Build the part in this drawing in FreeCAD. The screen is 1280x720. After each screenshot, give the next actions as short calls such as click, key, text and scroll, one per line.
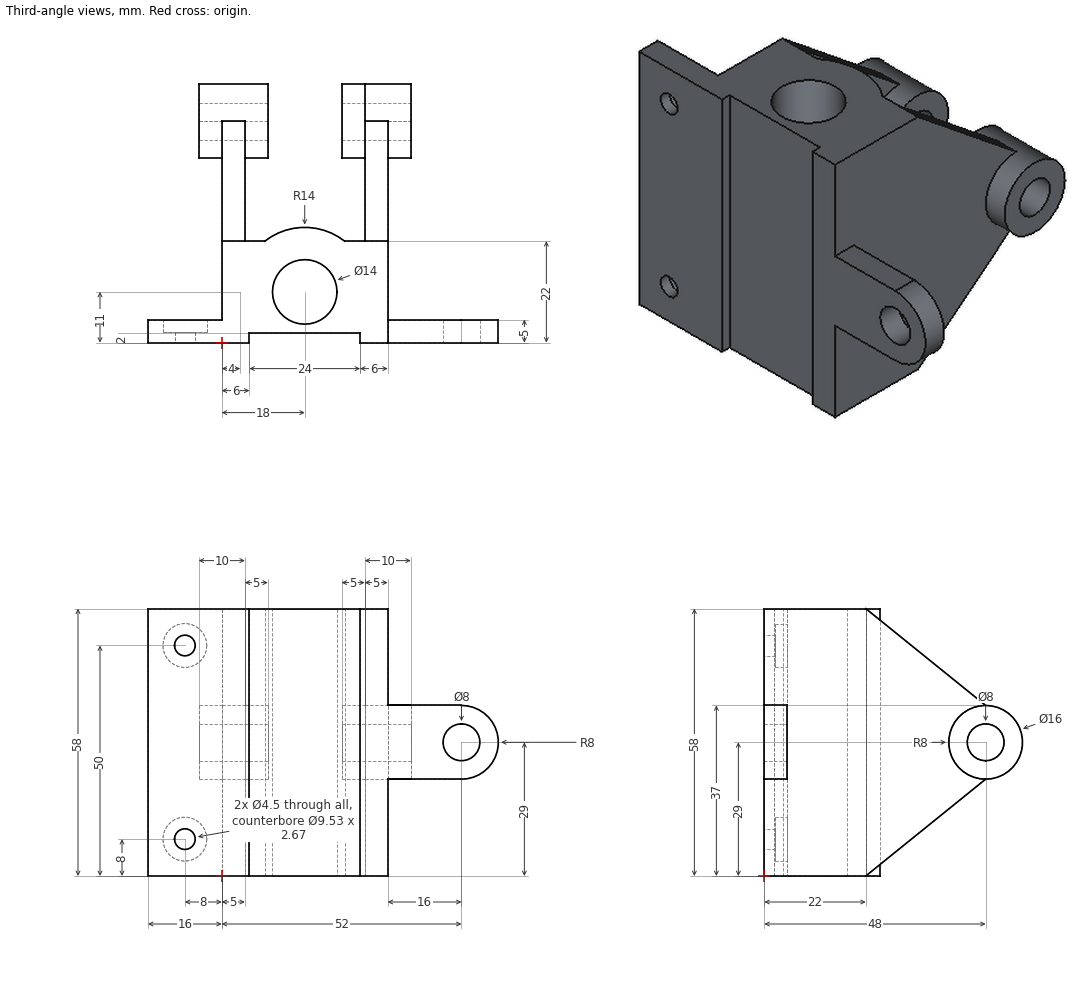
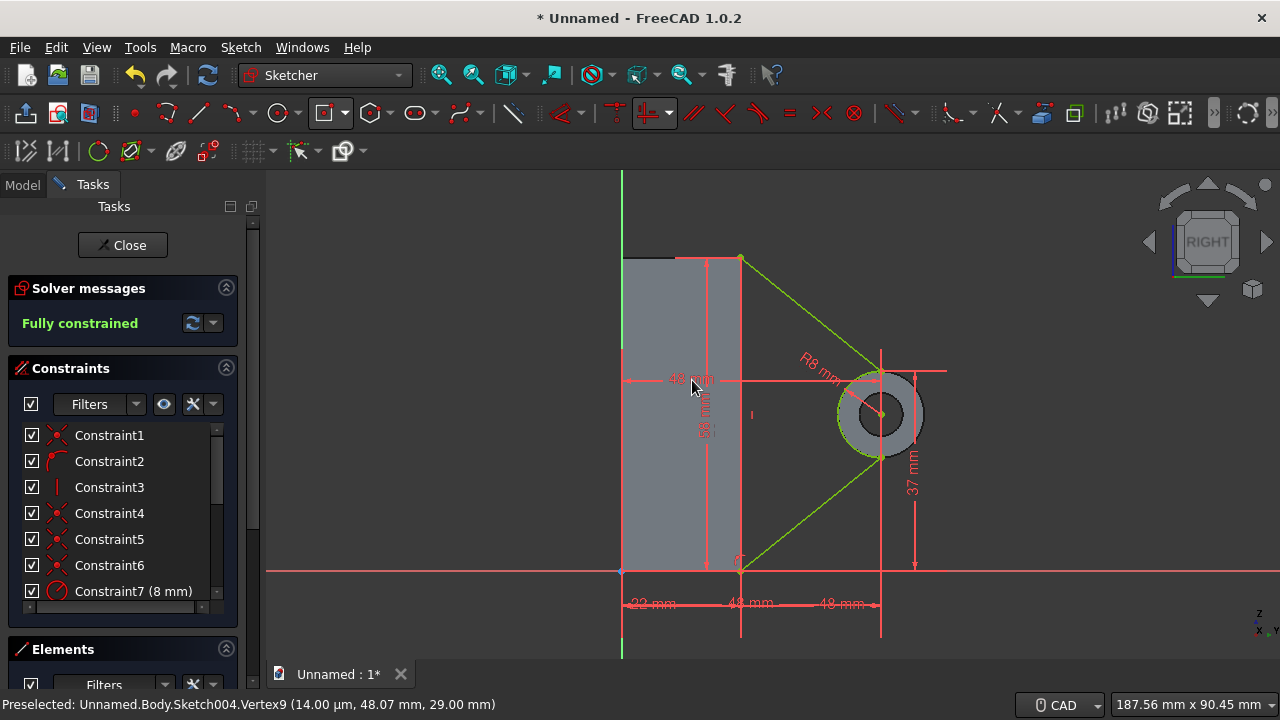
click(123, 245)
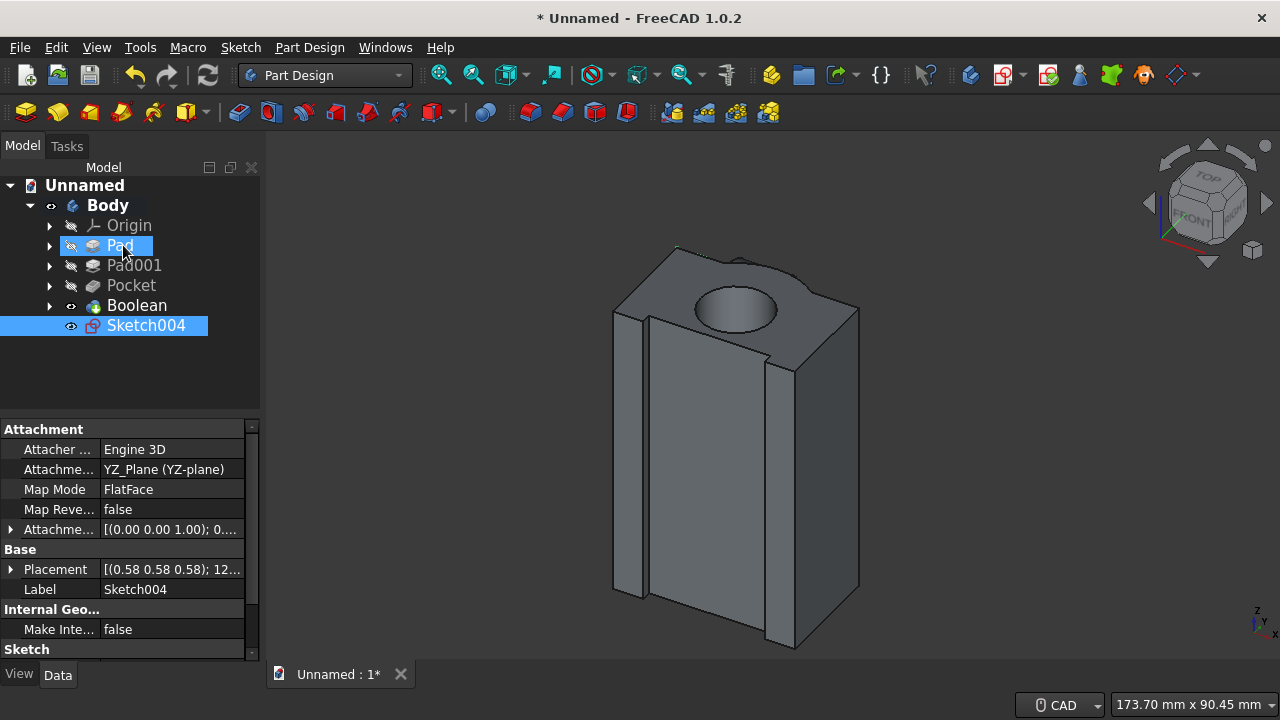
click(26, 112)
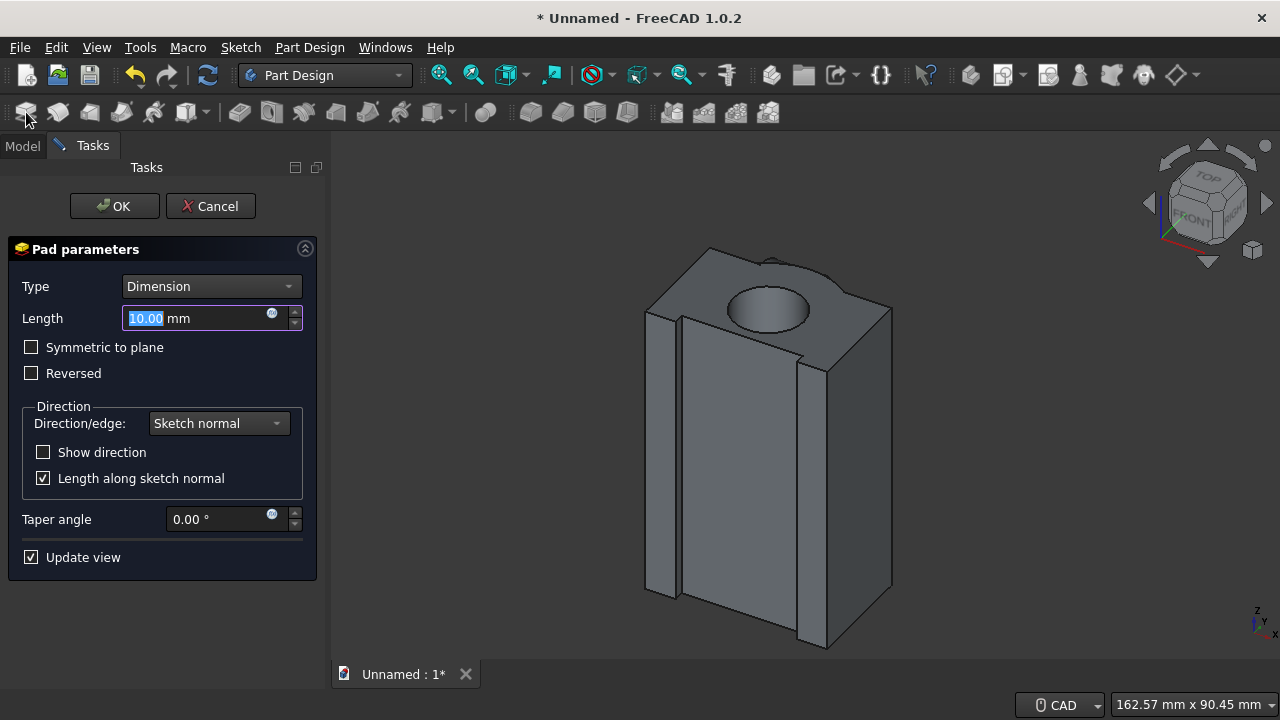
text(5)
key(Tab)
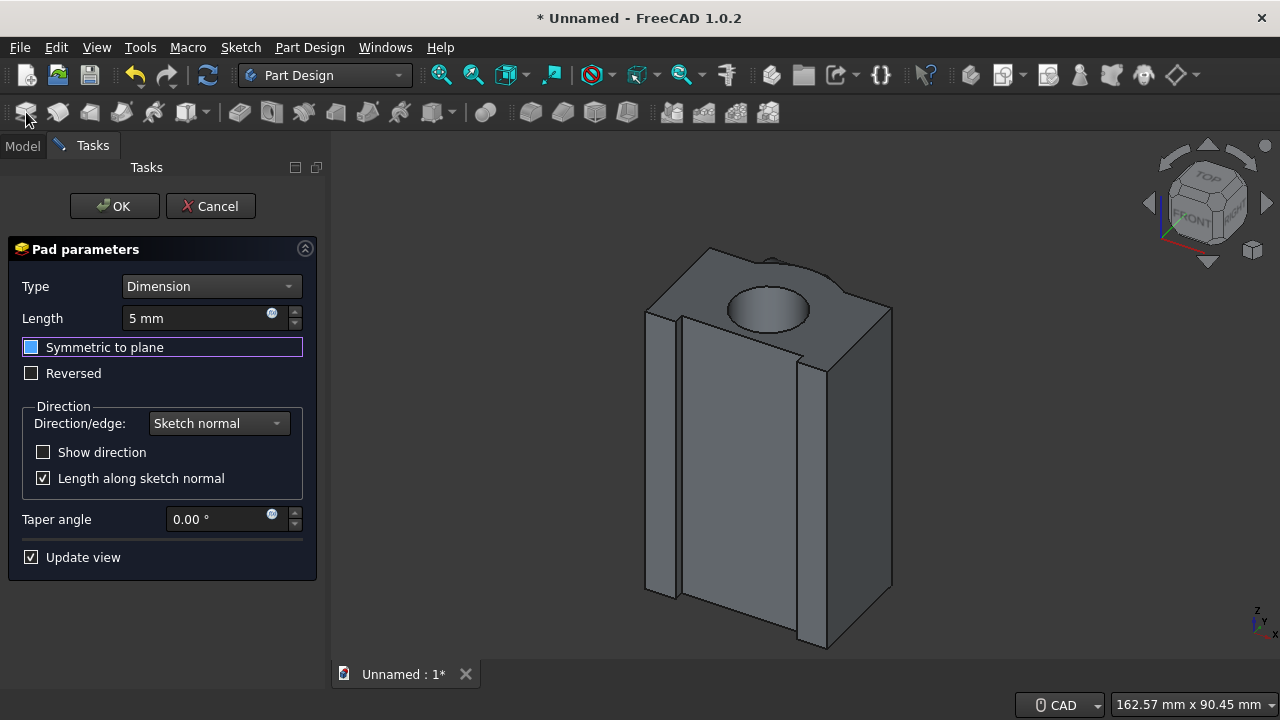
click(115, 206)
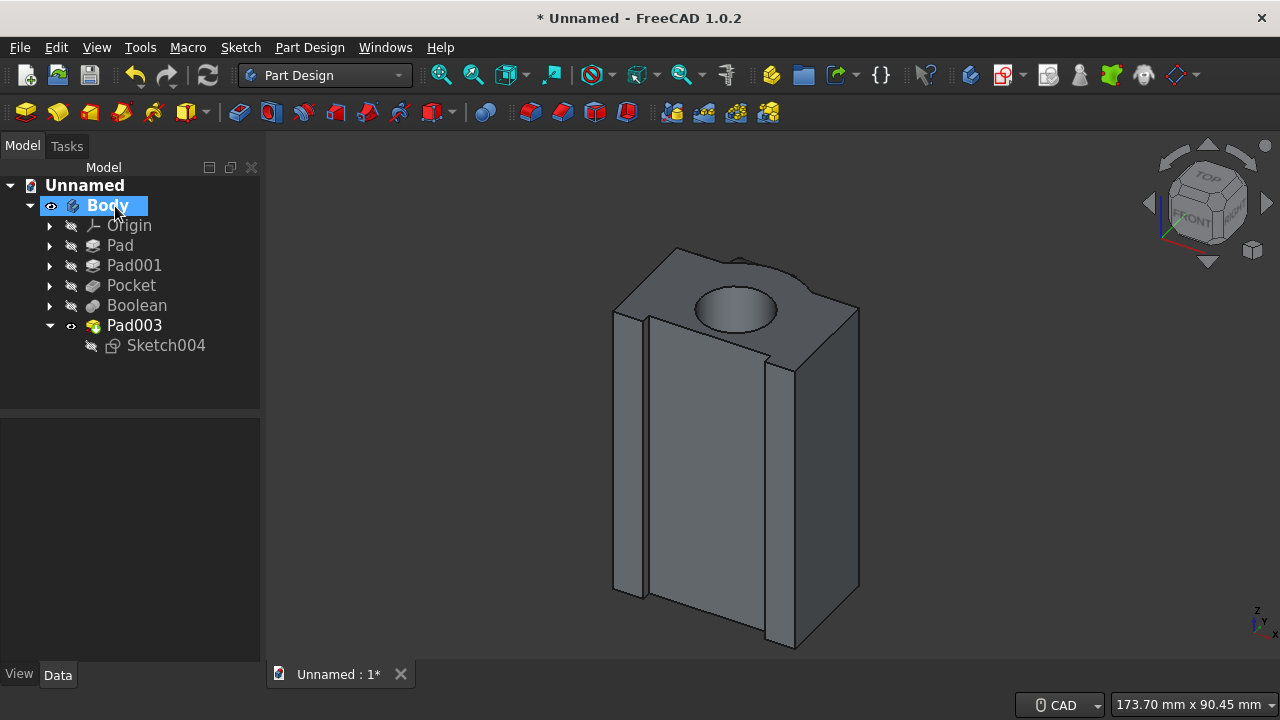
click(50, 226)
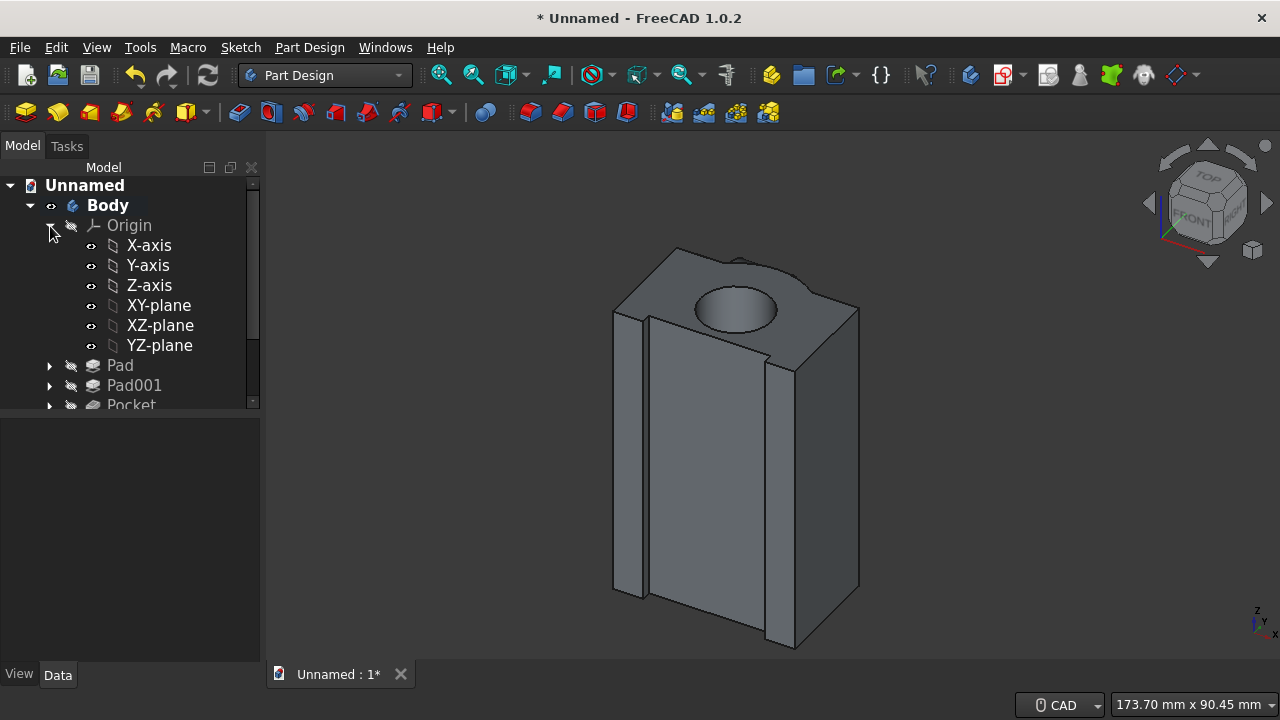
click(136, 346)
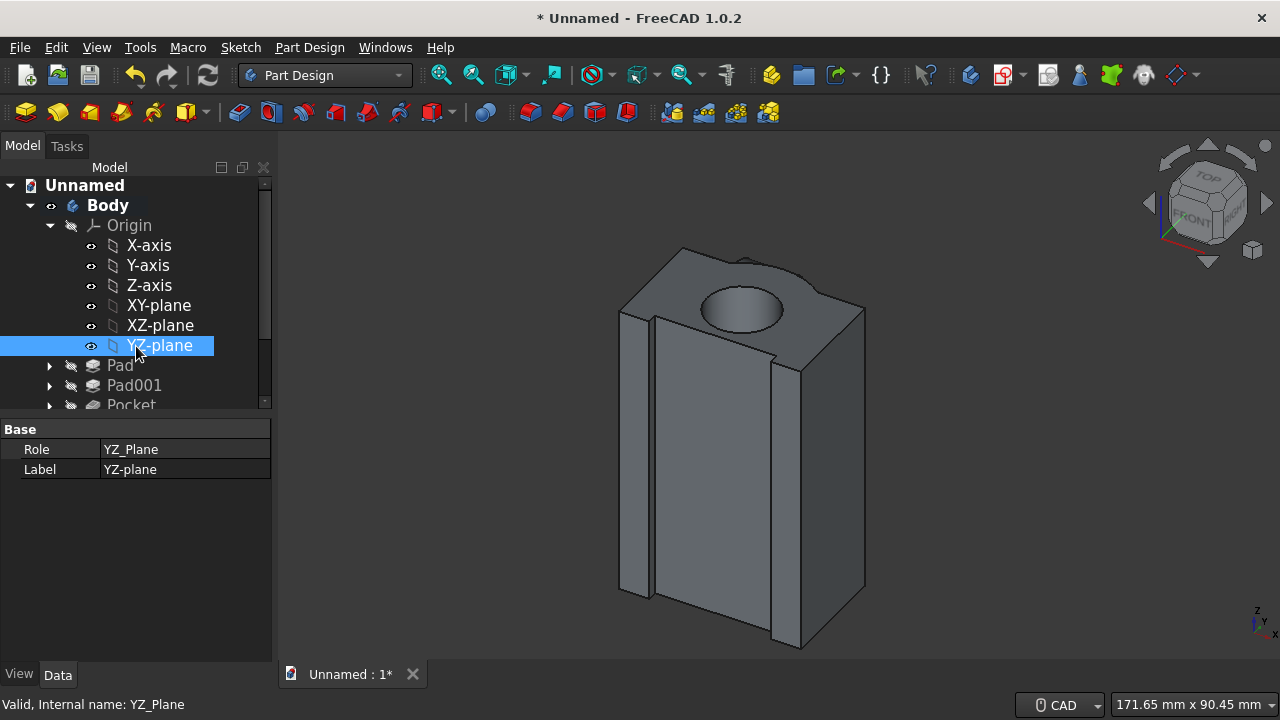
click(1176, 76)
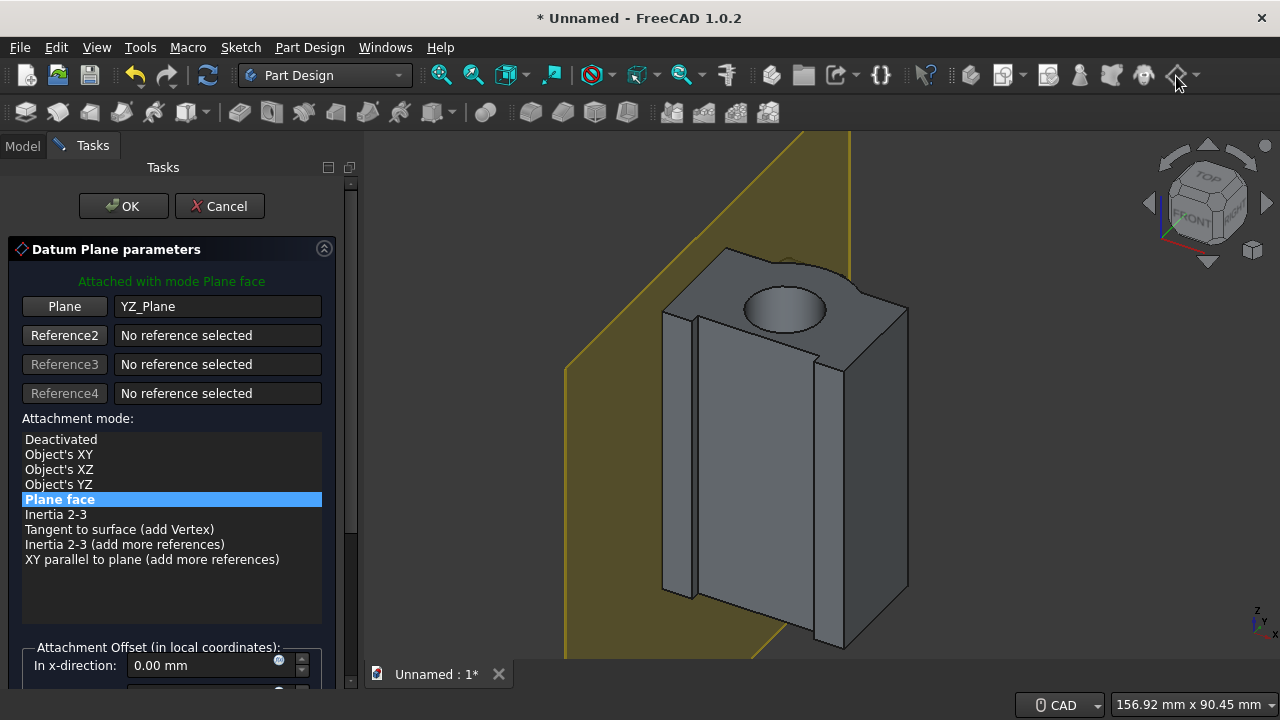
scroll(351, 432, down, 2)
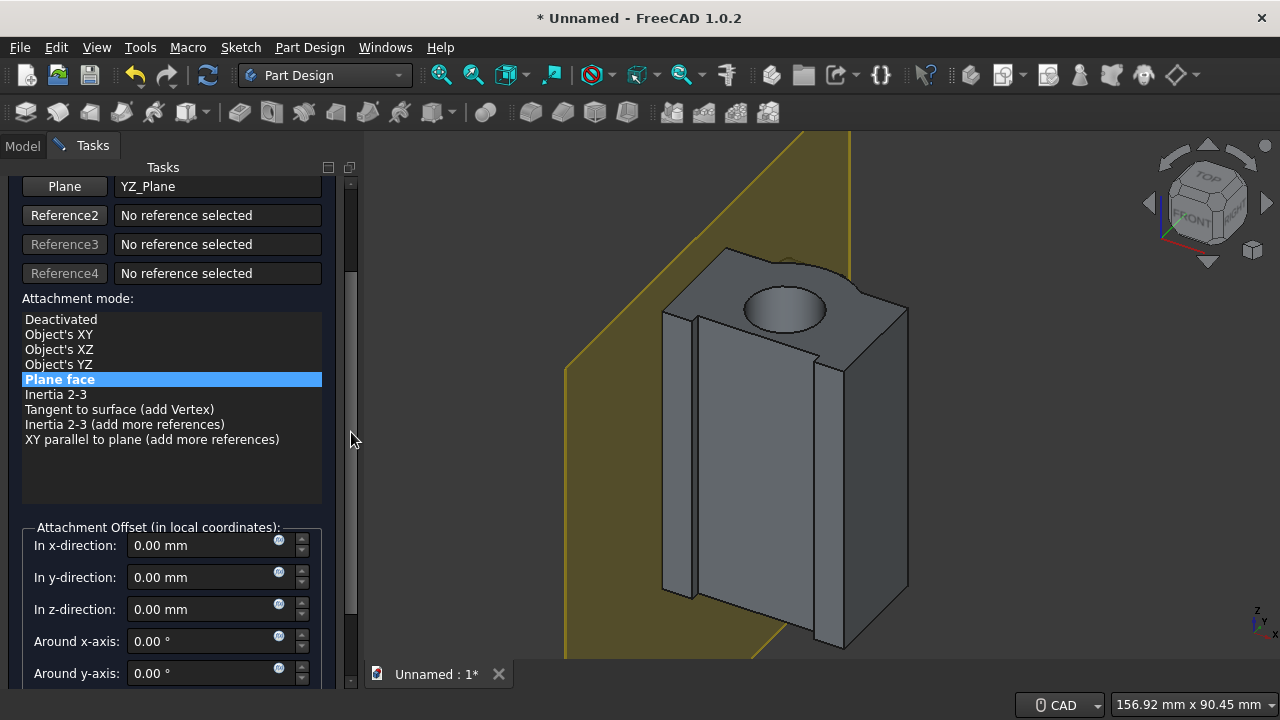
triple_click(210, 609)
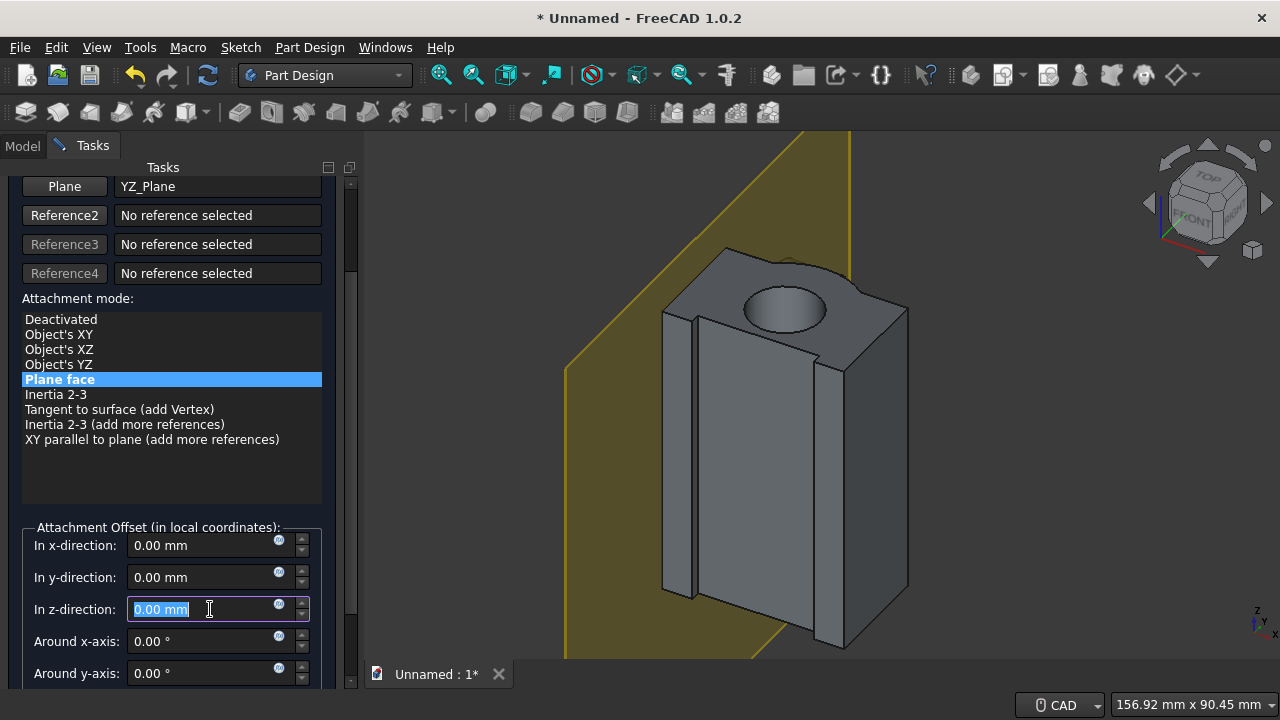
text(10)
key(Tab)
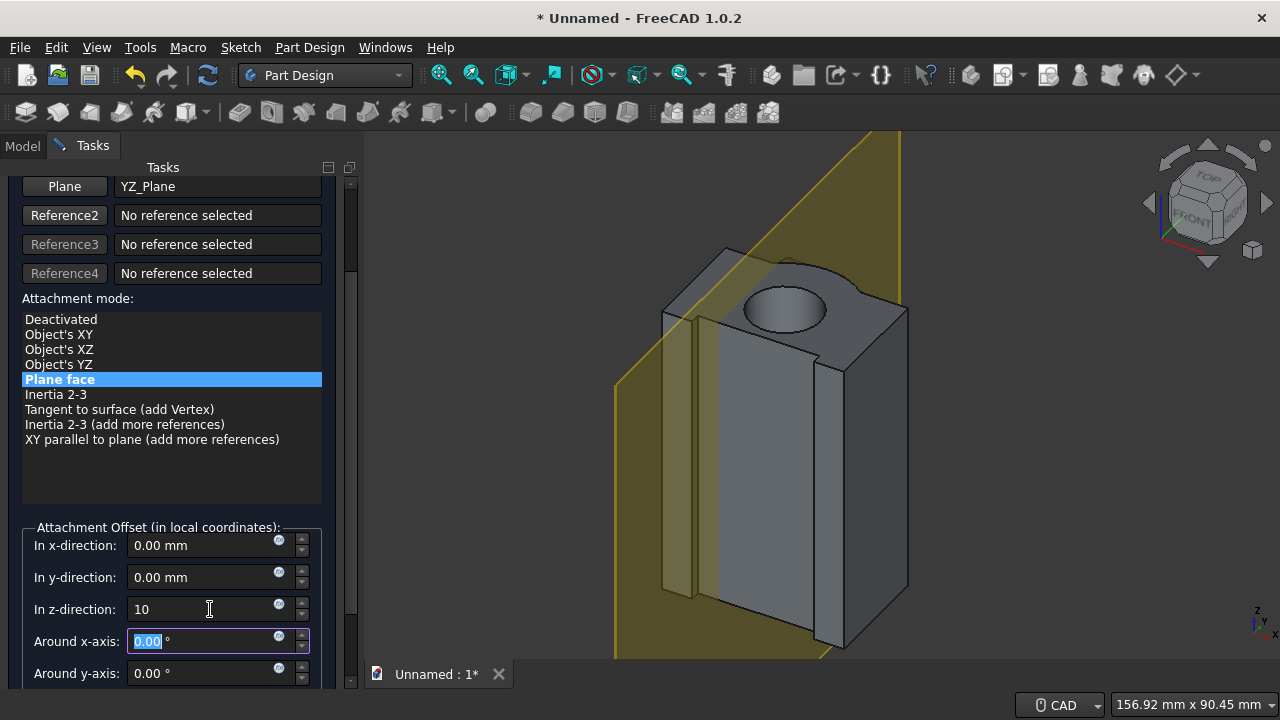
scroll(351, 432, up, 3)